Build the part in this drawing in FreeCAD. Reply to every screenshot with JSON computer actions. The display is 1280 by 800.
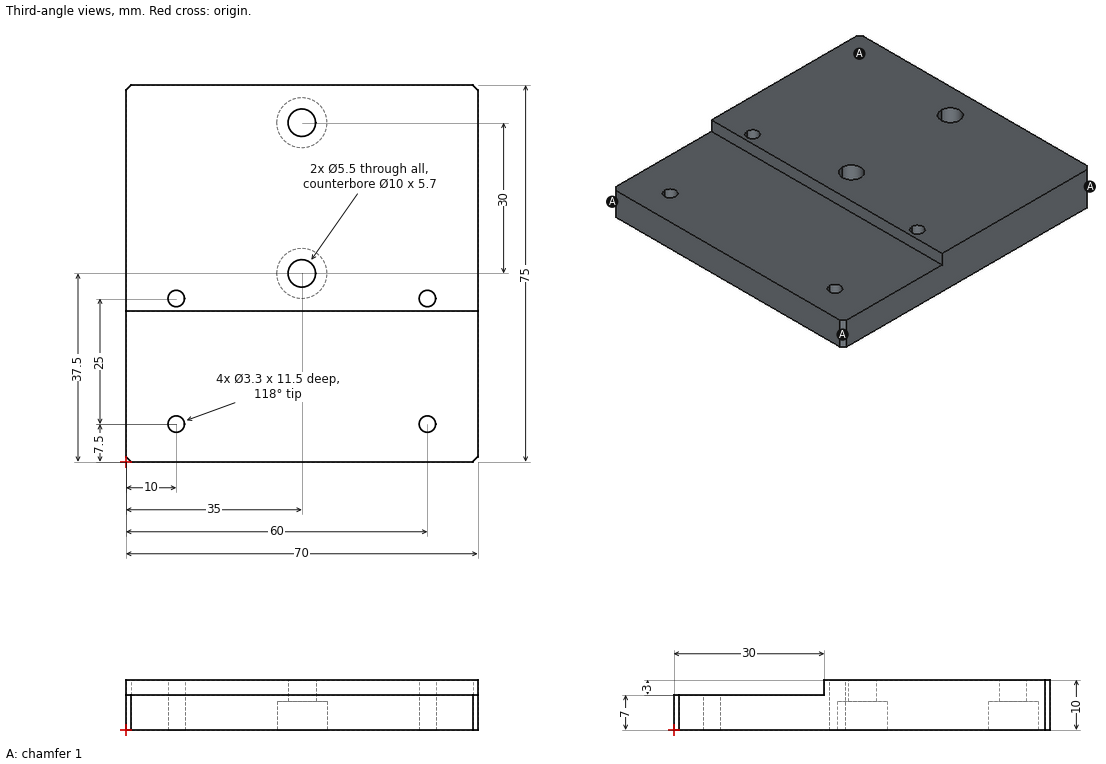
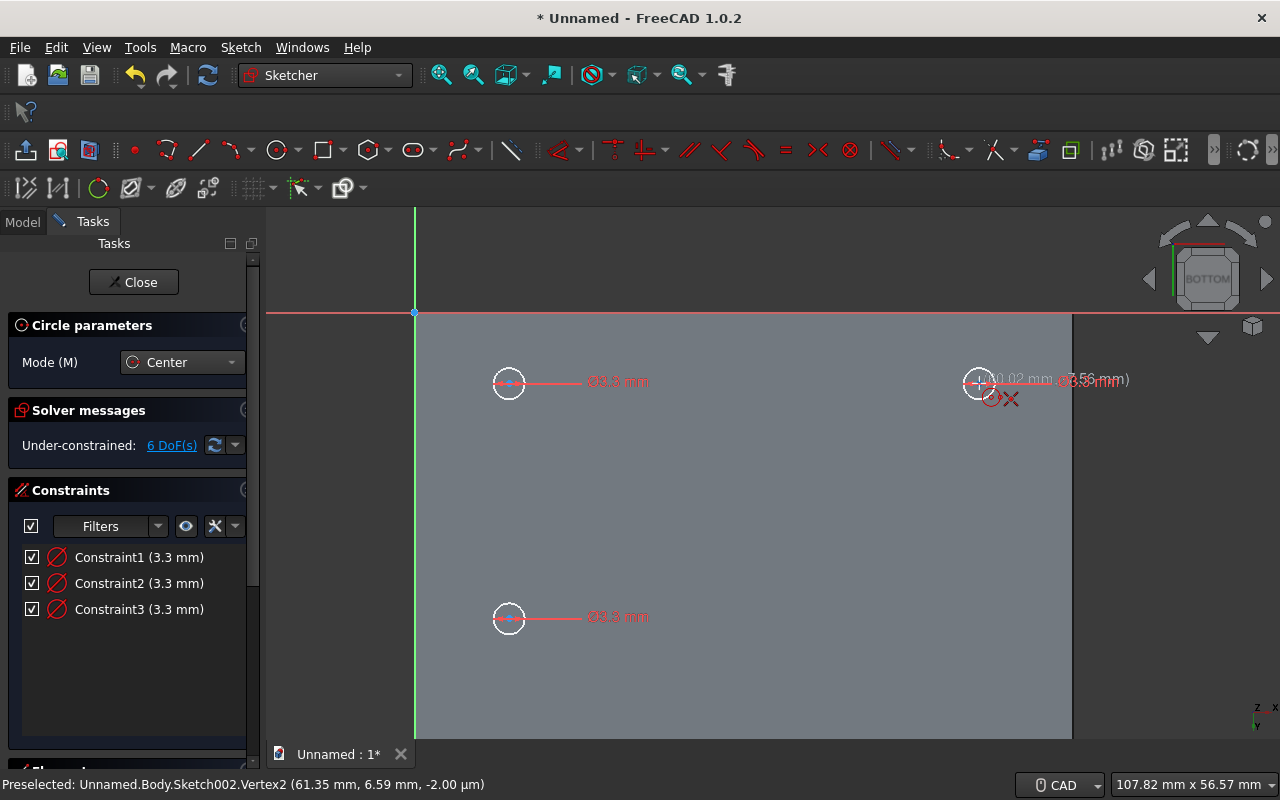
{"action": "scroll", "coordinate": [979, 618], "scroll_direction": "up", "scroll_amount": 2}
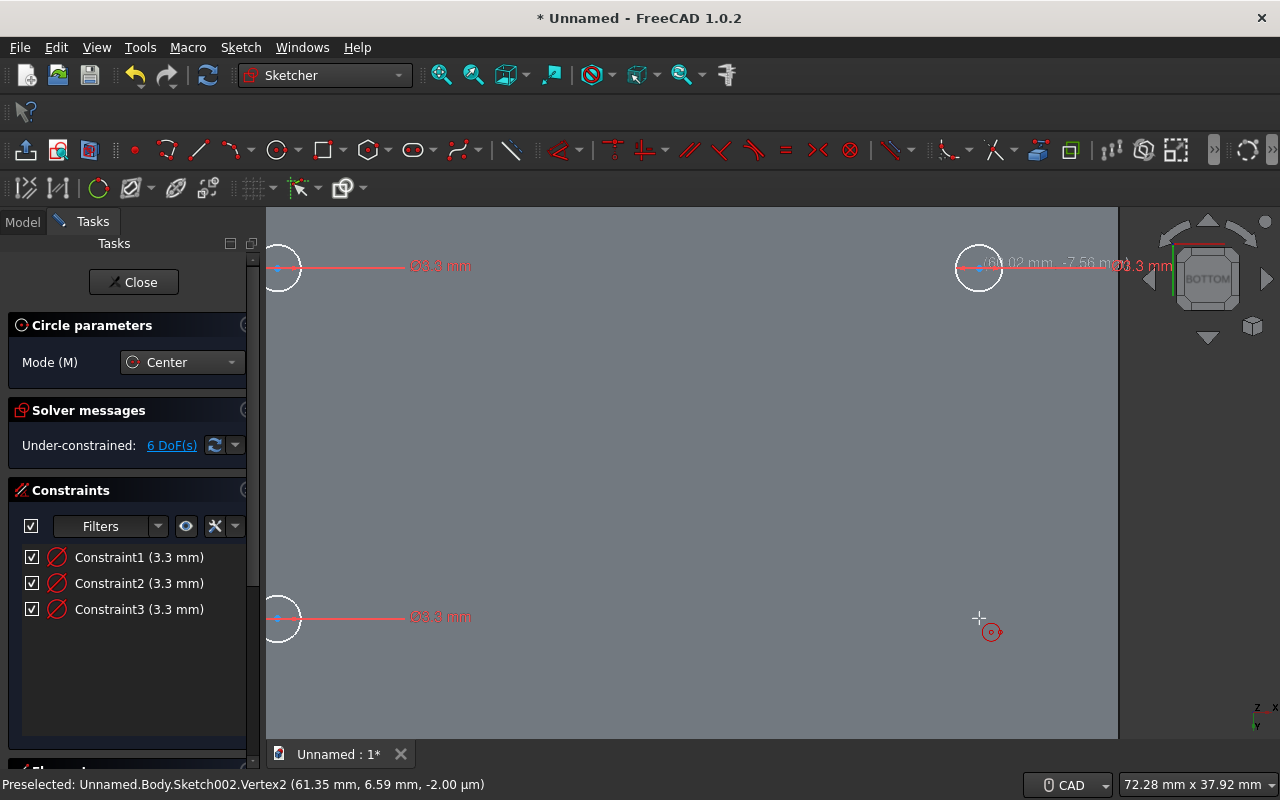
{"action": "left_click", "coordinate": [979, 618]}
{"action": "mouse_move", "coordinate": [995, 602]}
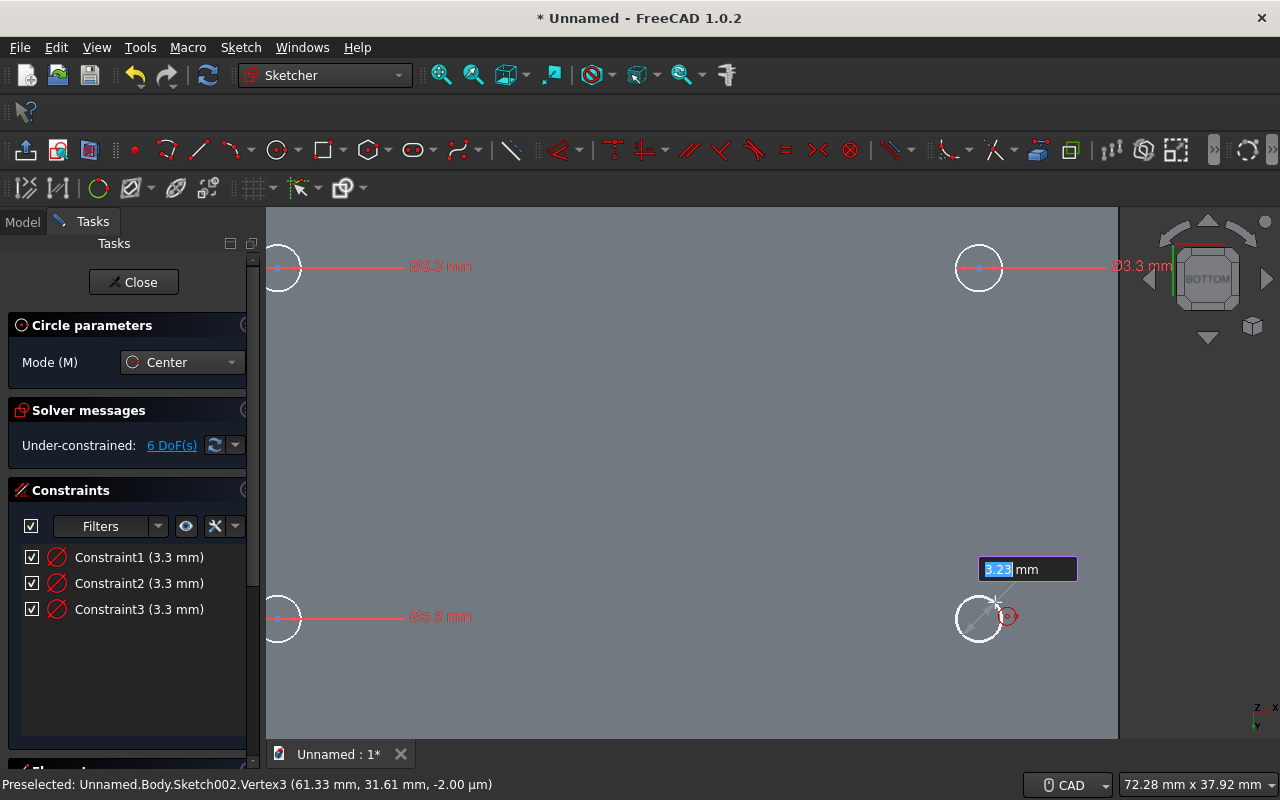
{"action": "type", "text": "3.3"}
{"action": "key", "text": "Return"}
{"action": "key", "text": "Escape"}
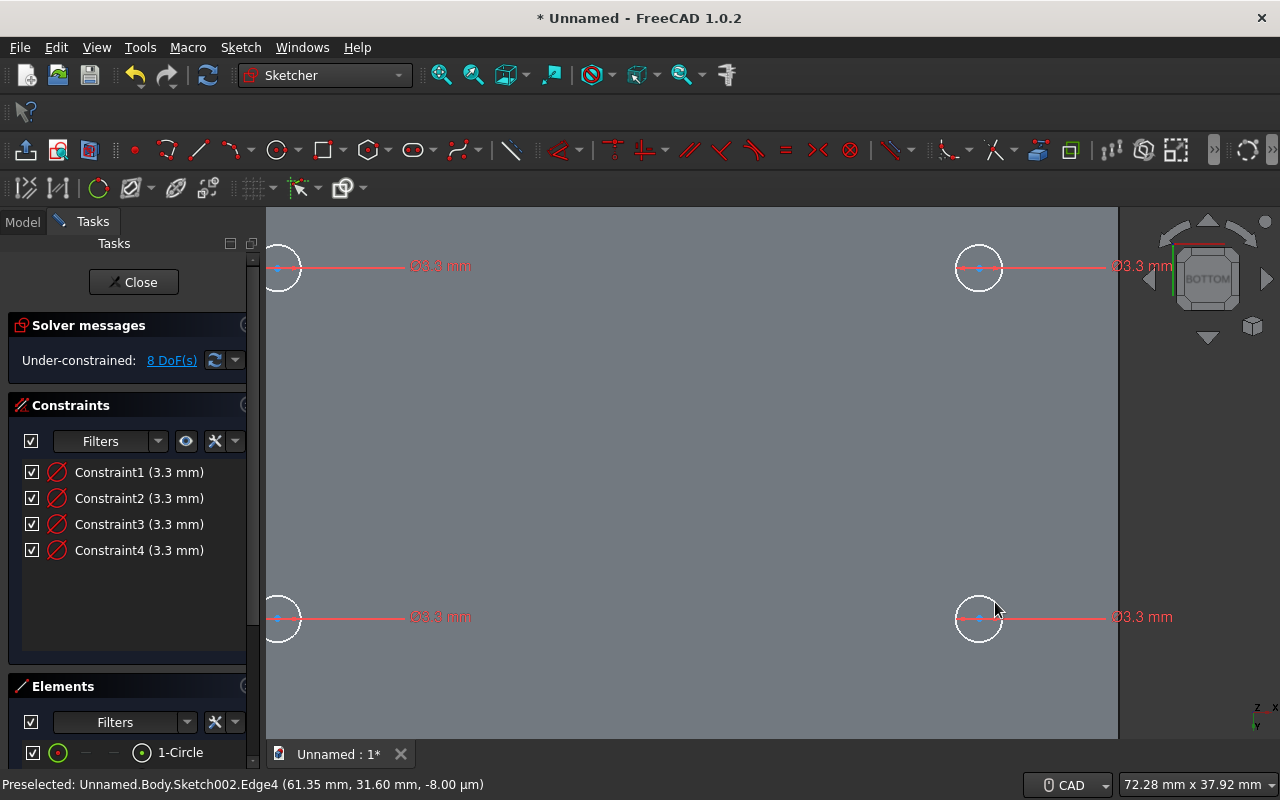
{"action": "scroll", "coordinate": [979, 618], "scroll_direction": "down", "scroll_amount": 2}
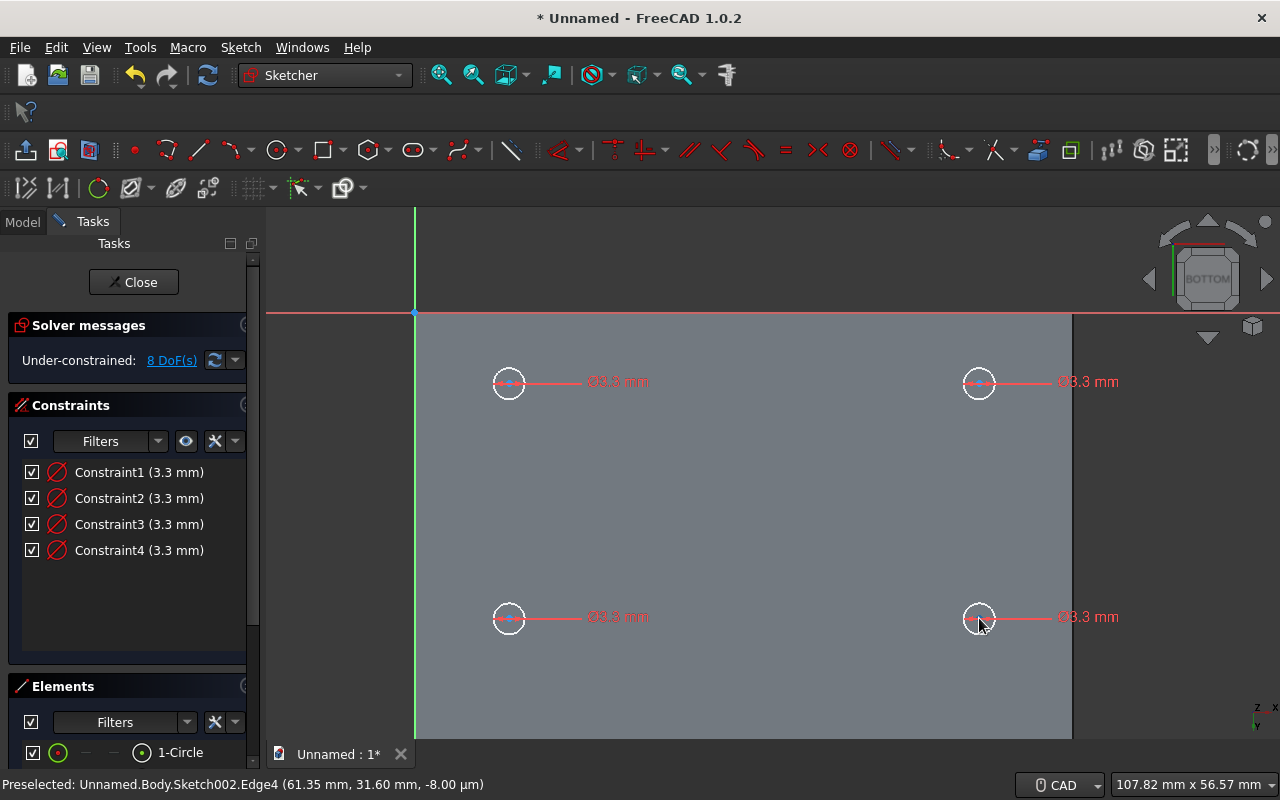
{"action": "left_click", "coordinate": [509, 384]}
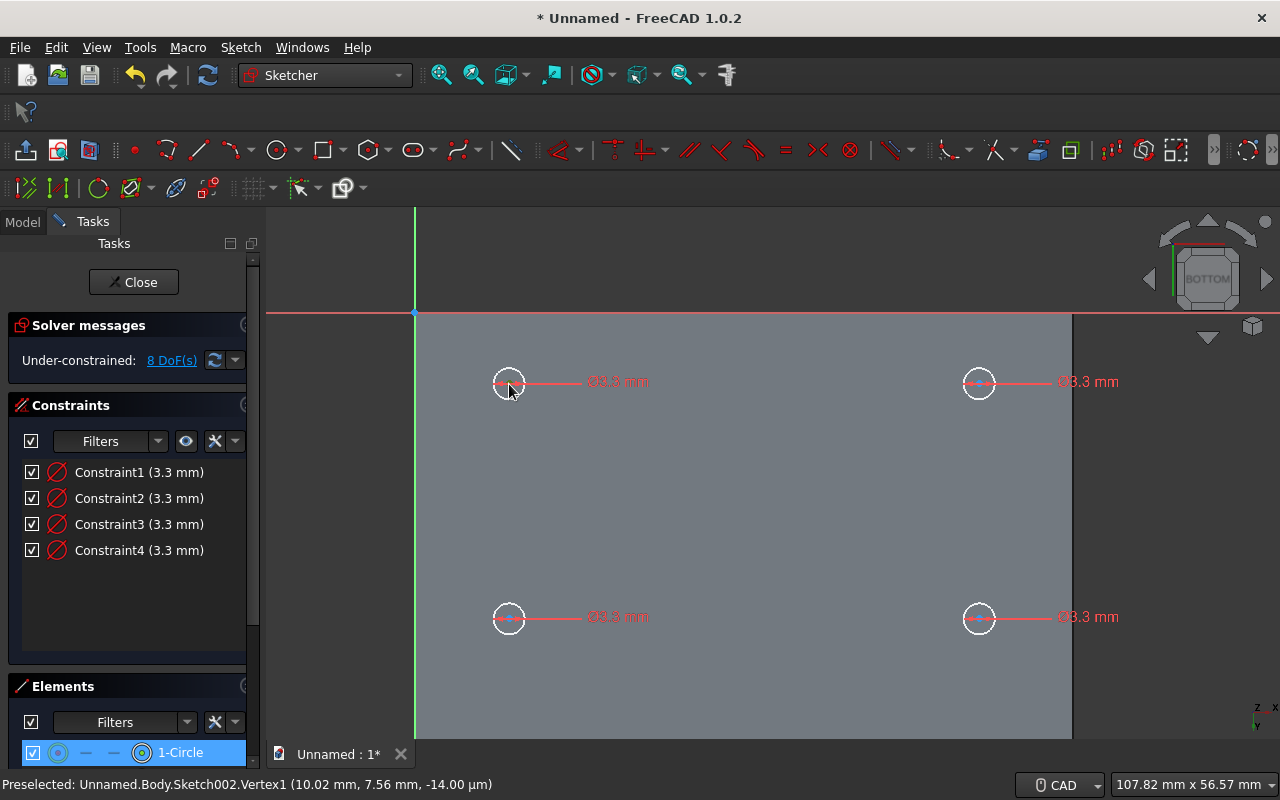
{"action": "left_click", "coordinate": [509, 619]}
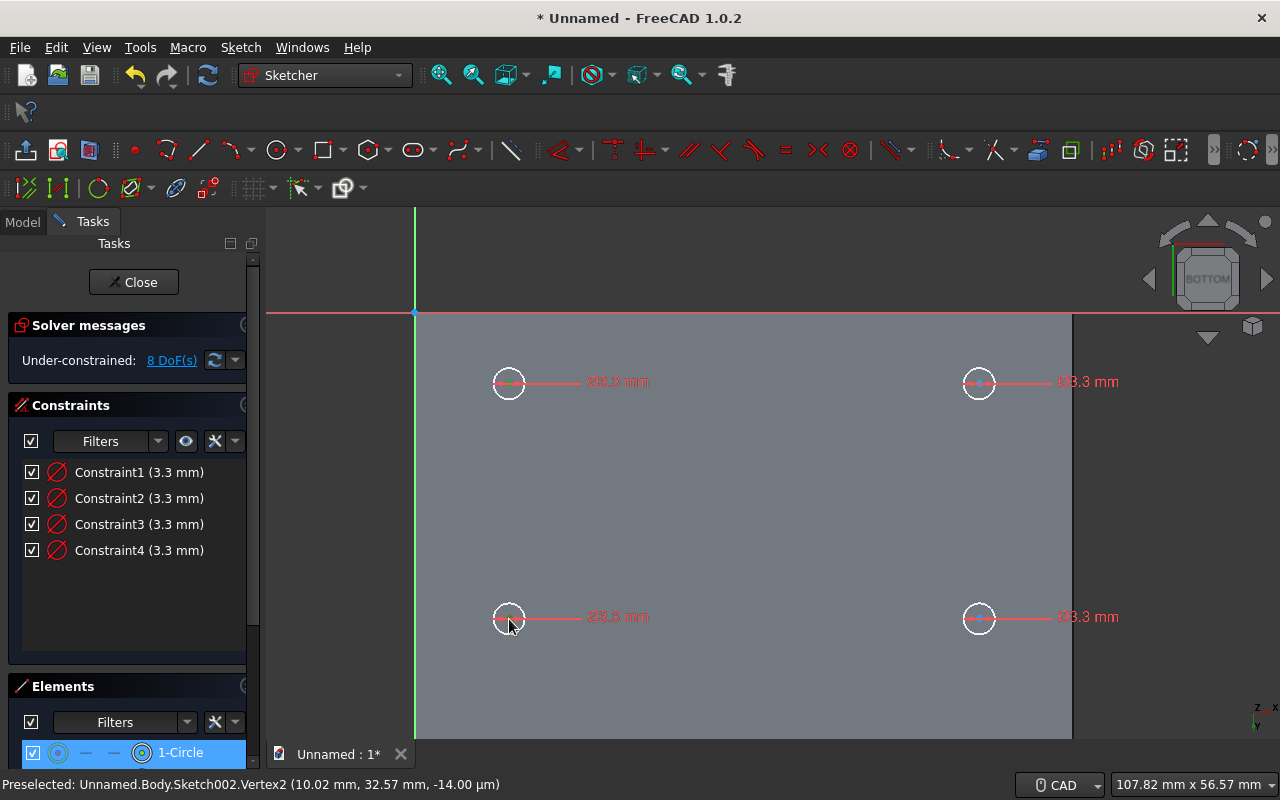
{"action": "left_click", "coordinate": [668, 150]}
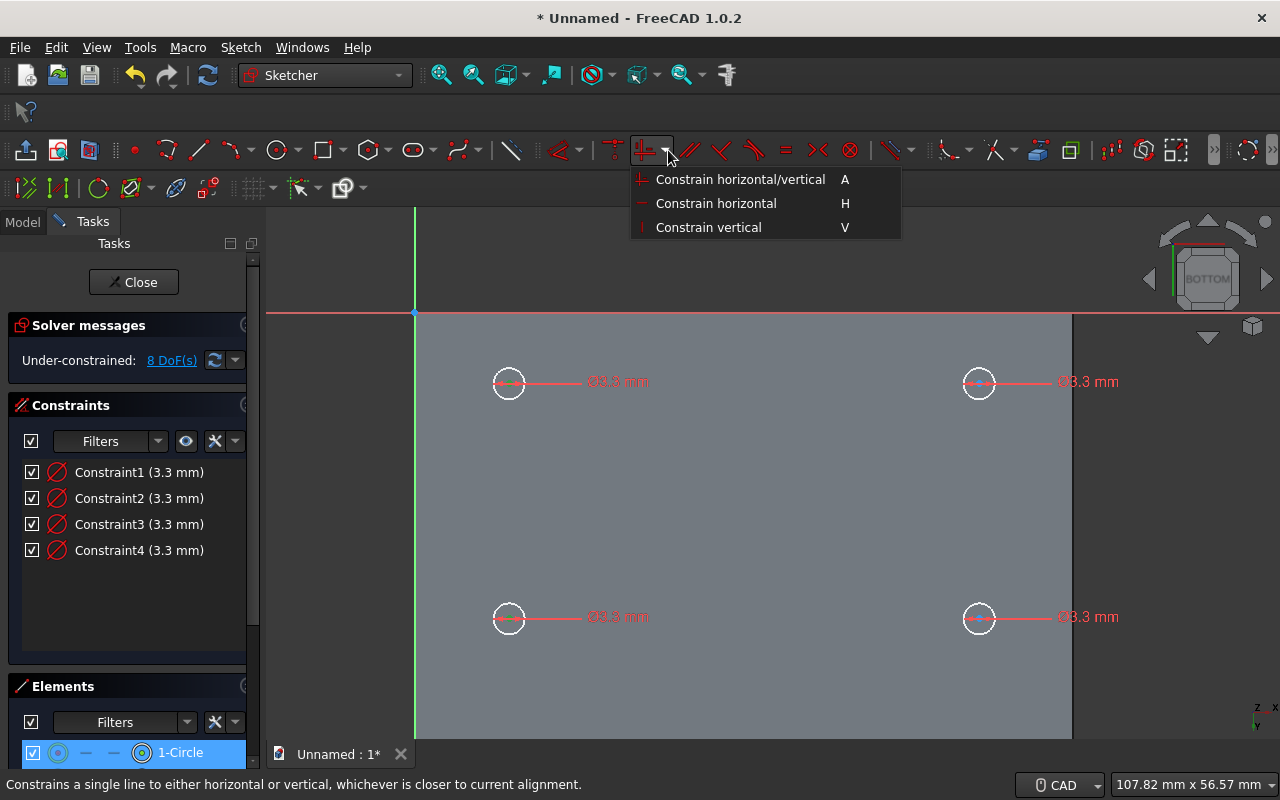
{"action": "left_click", "coordinate": [766, 227]}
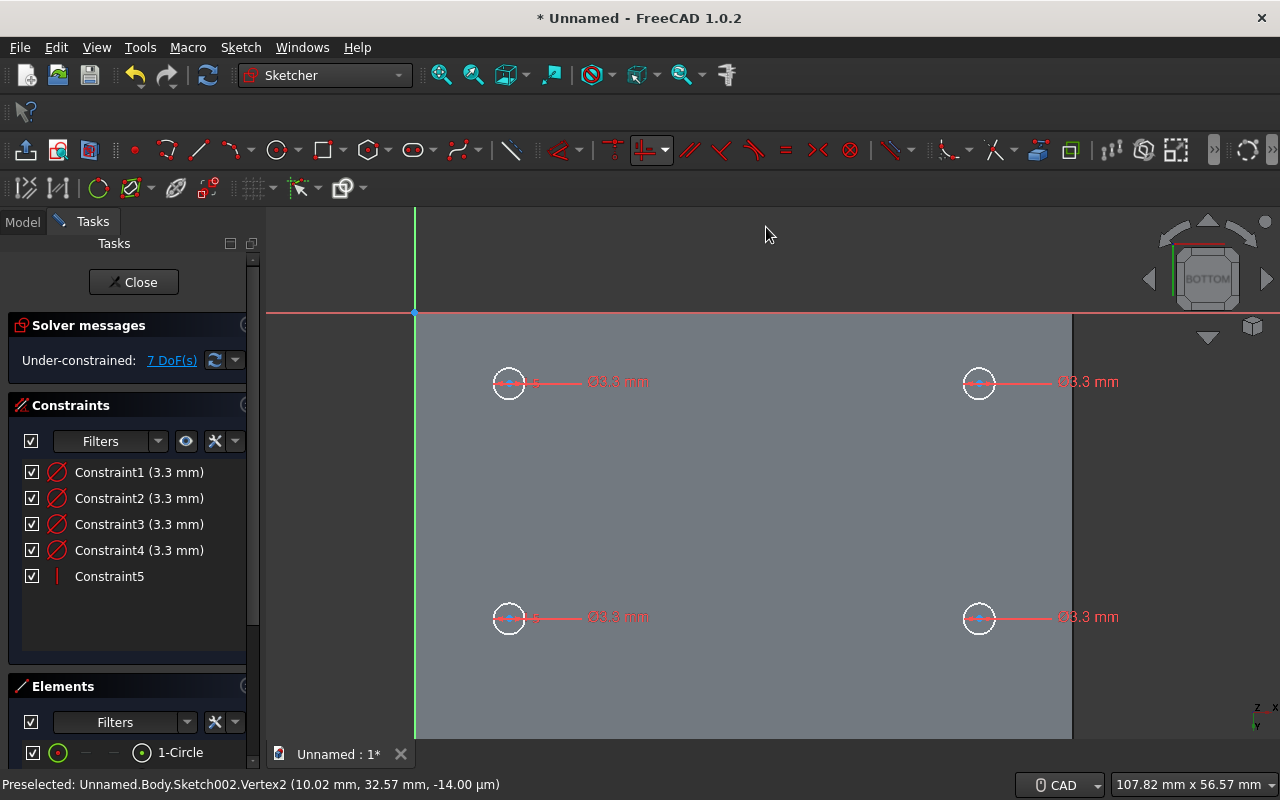
{"action": "left_click", "coordinate": [509, 384]}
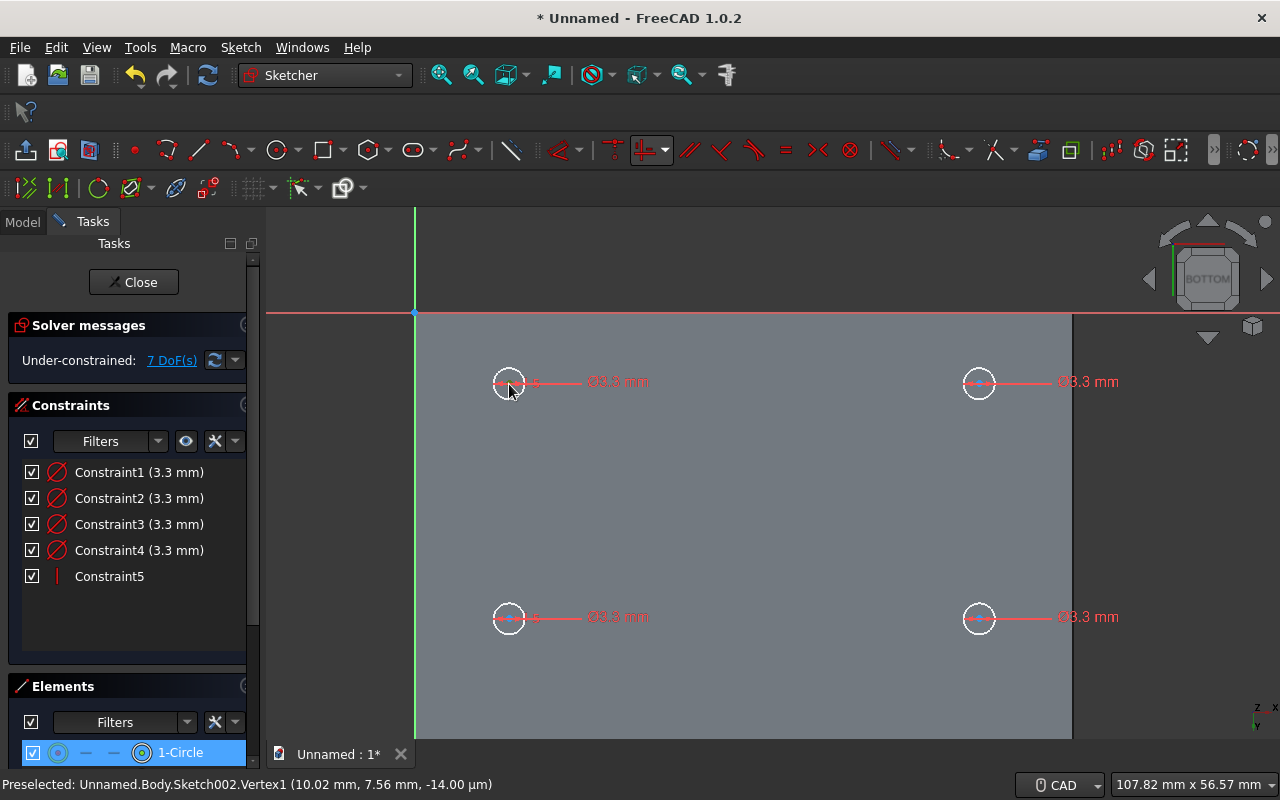
{"action": "left_click", "coordinate": [979, 384]}